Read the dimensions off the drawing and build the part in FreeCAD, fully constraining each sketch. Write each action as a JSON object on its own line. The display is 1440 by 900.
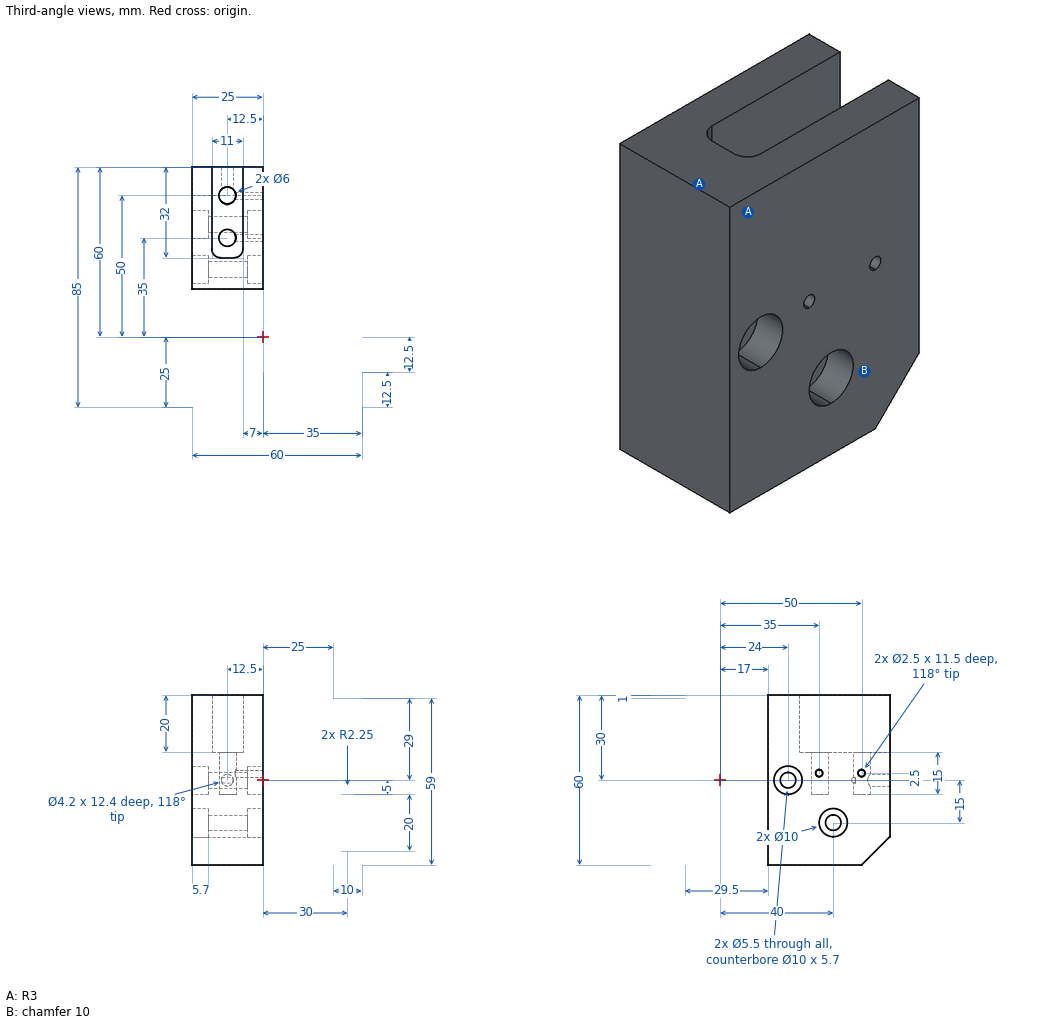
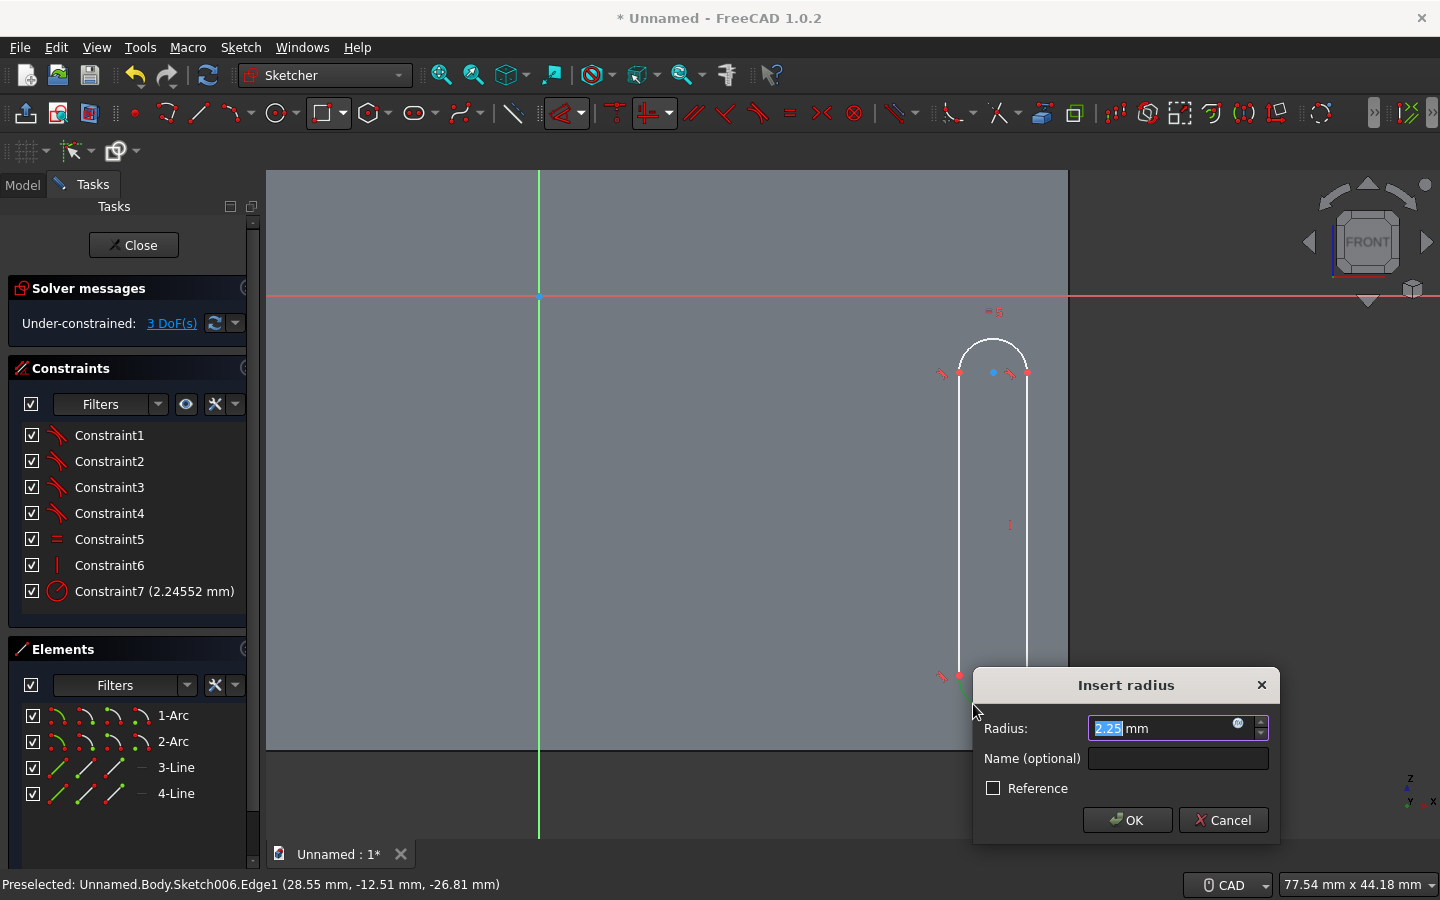
{"action": "type", "text": "2.25"}
{"action": "key", "text": "Return"}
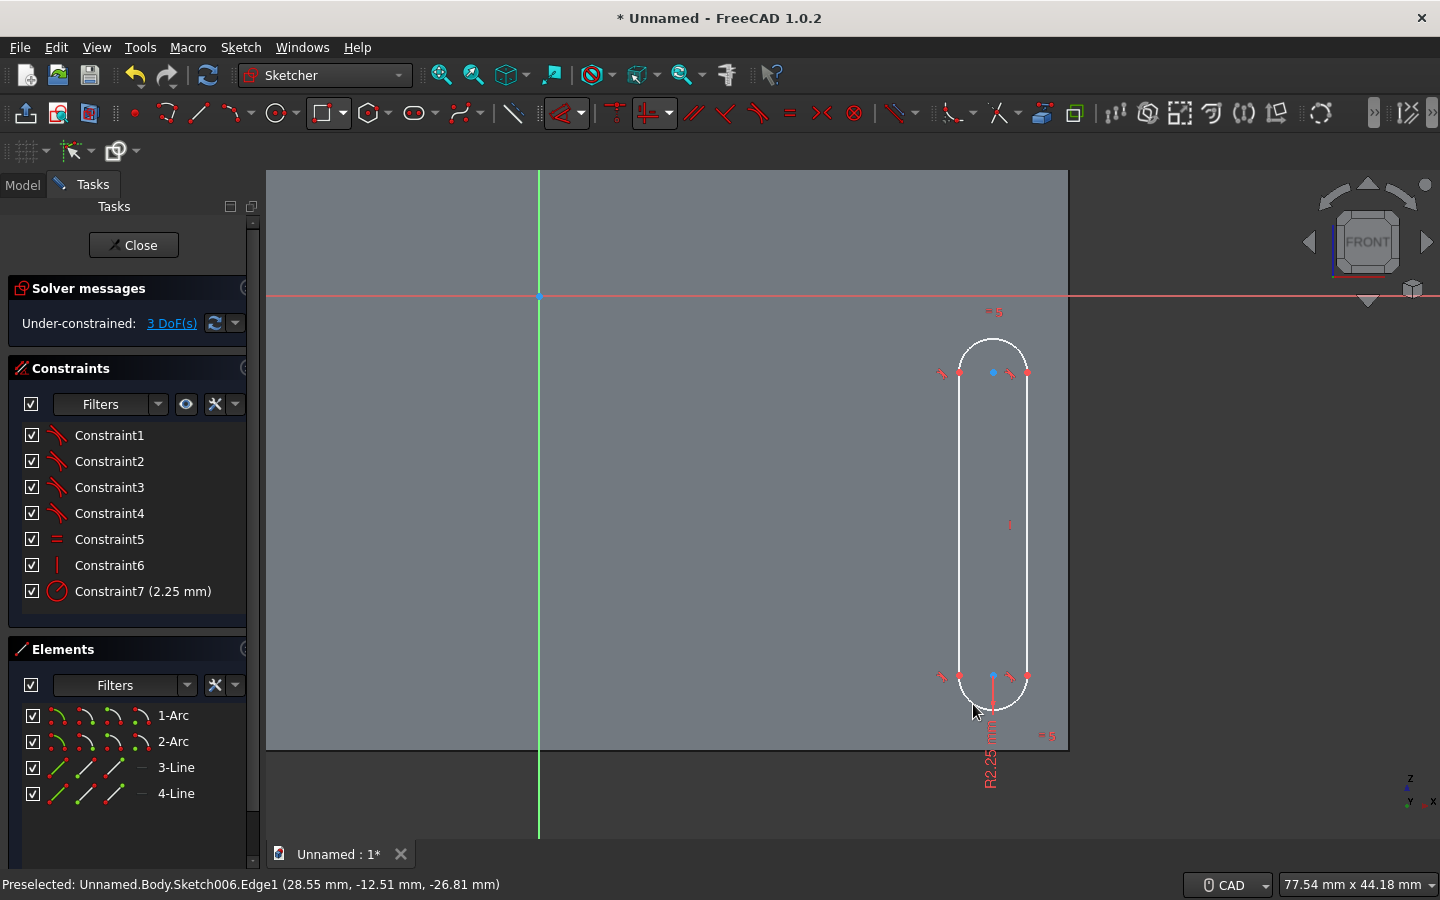
{"action": "left_click", "coordinate": [959, 585]}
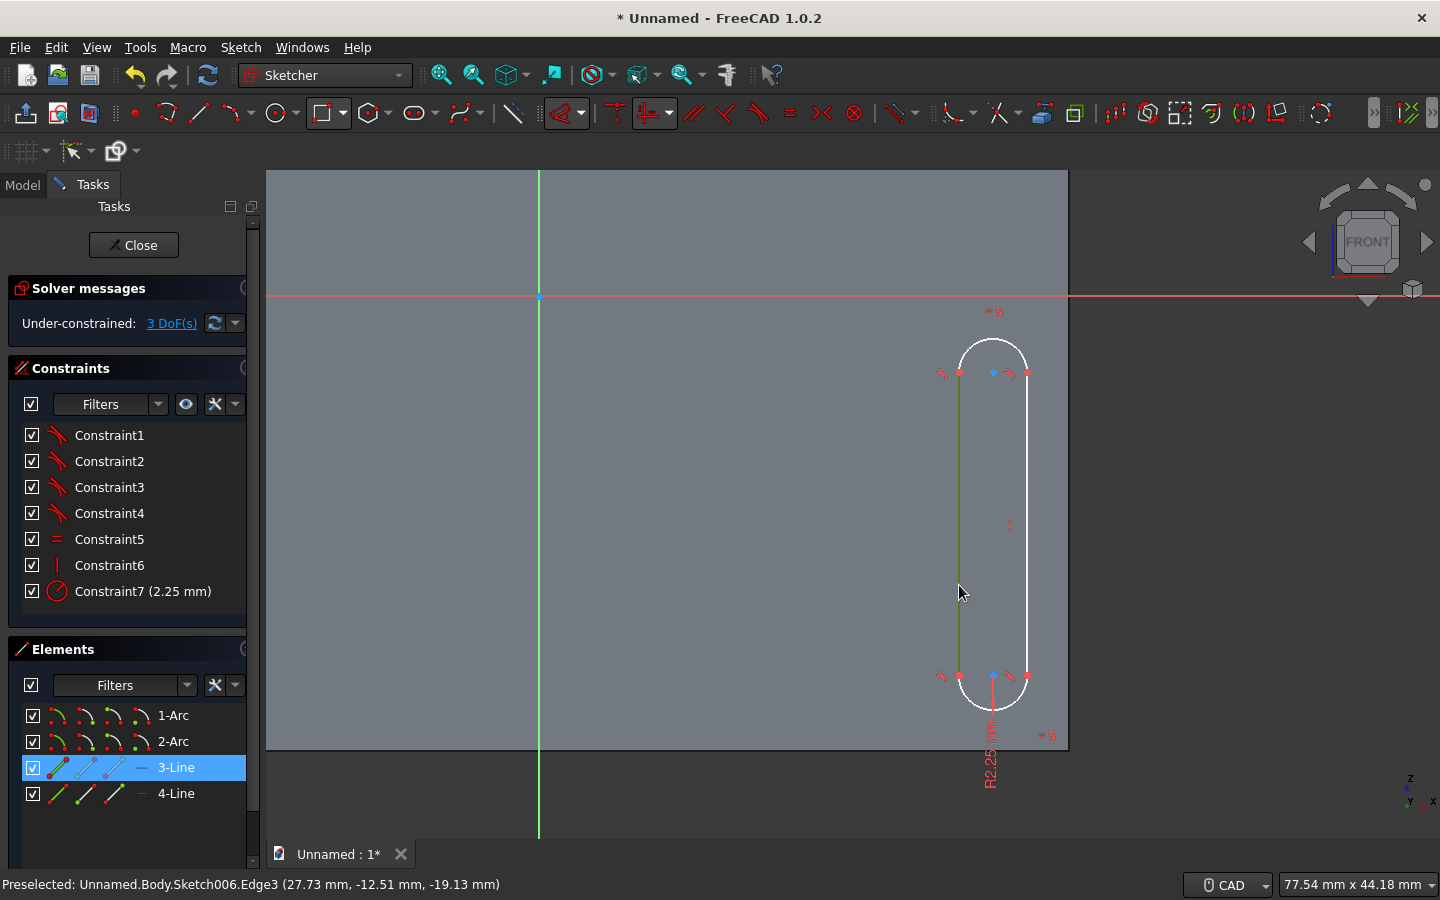
{"action": "key", "text": "i"}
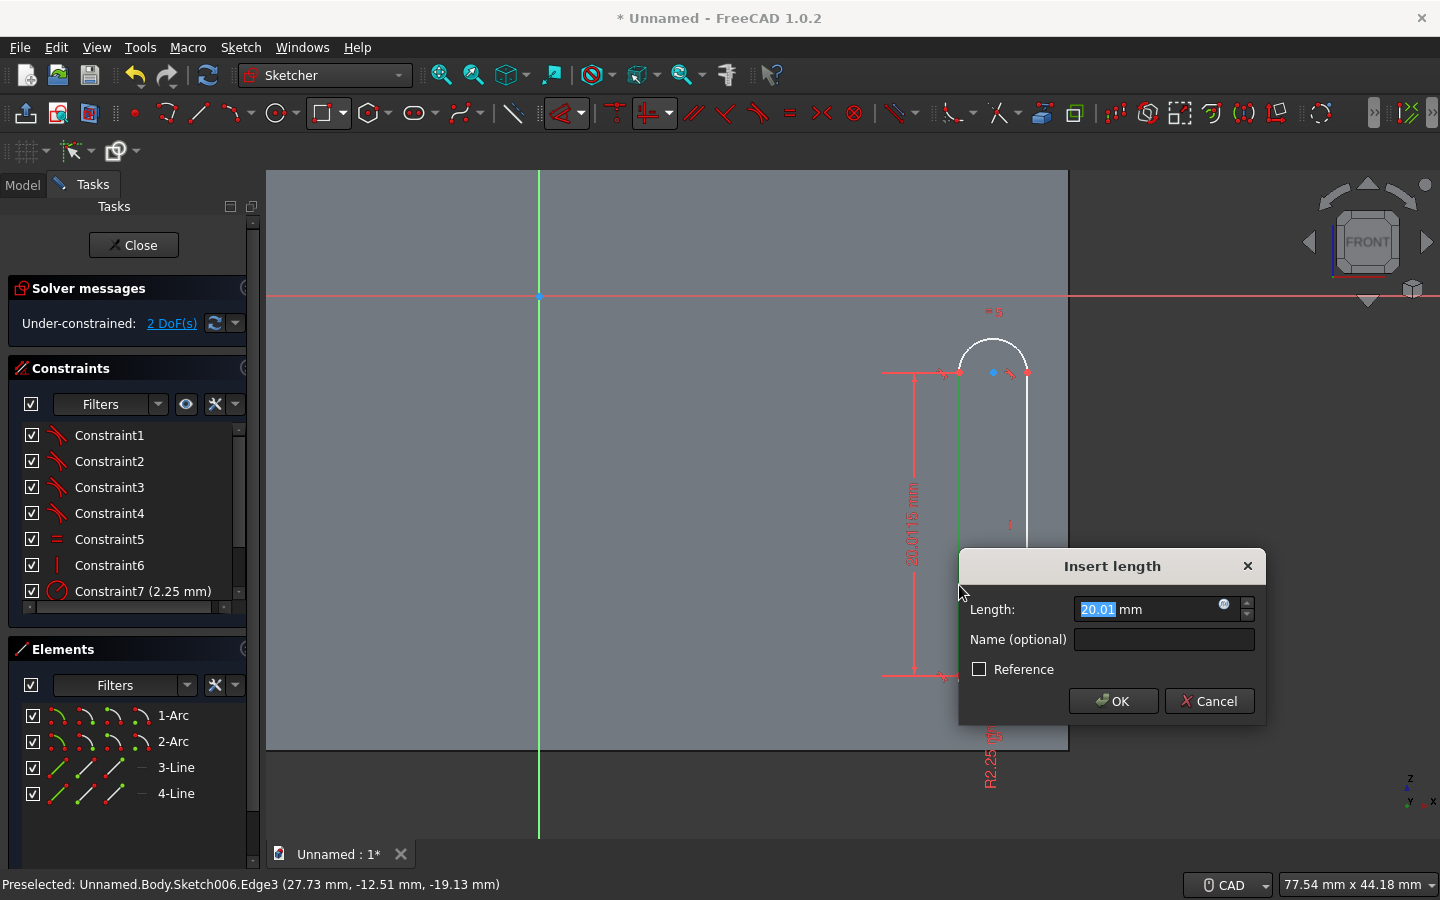
{"action": "type", "text": "20"}
{"action": "key", "text": "Return"}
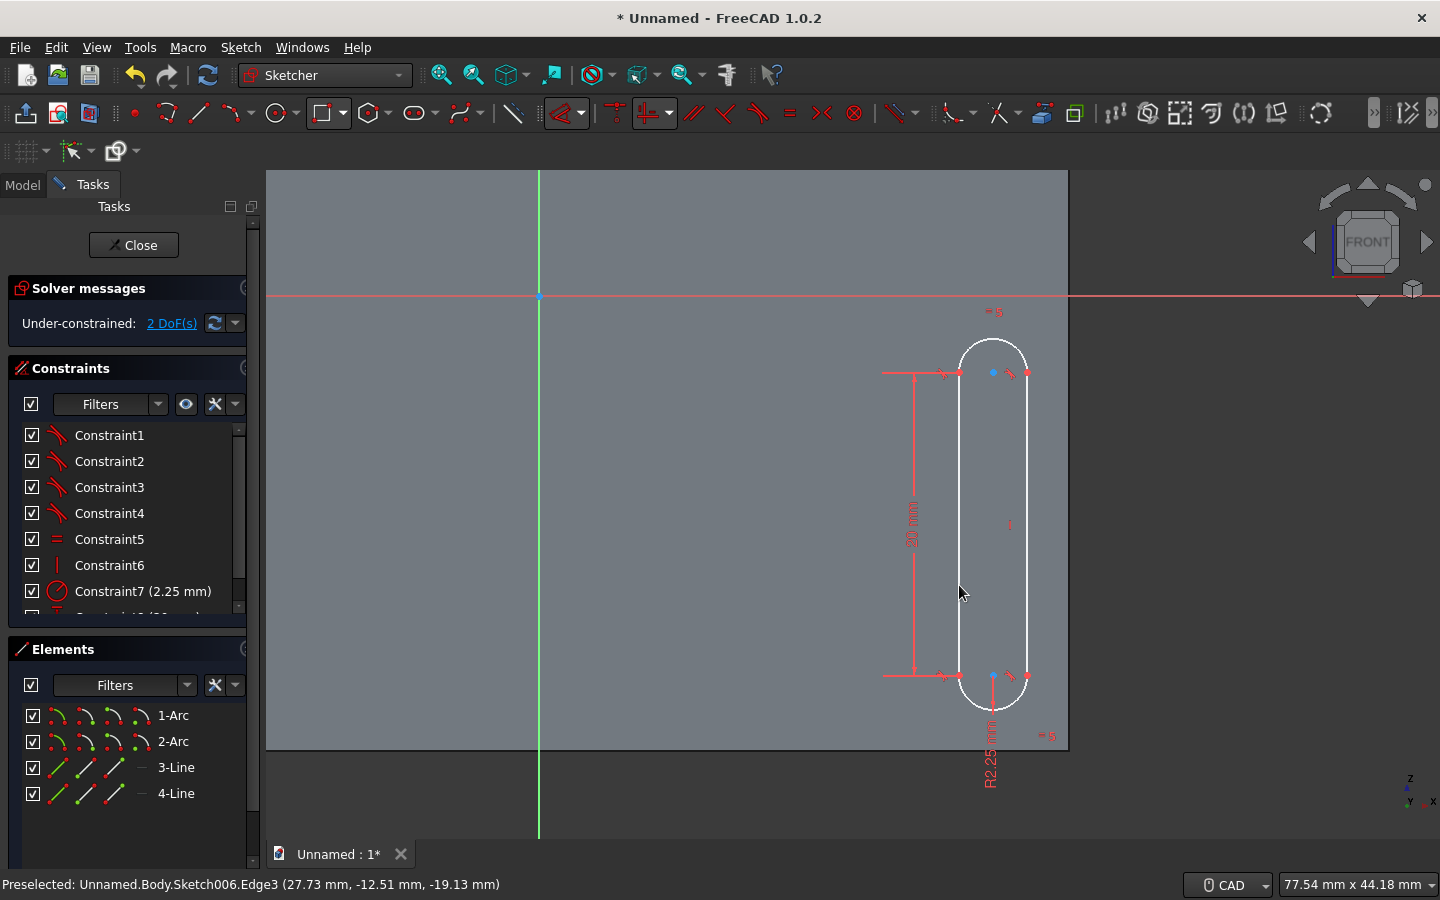
{"action": "left_click", "coordinate": [1027, 373]}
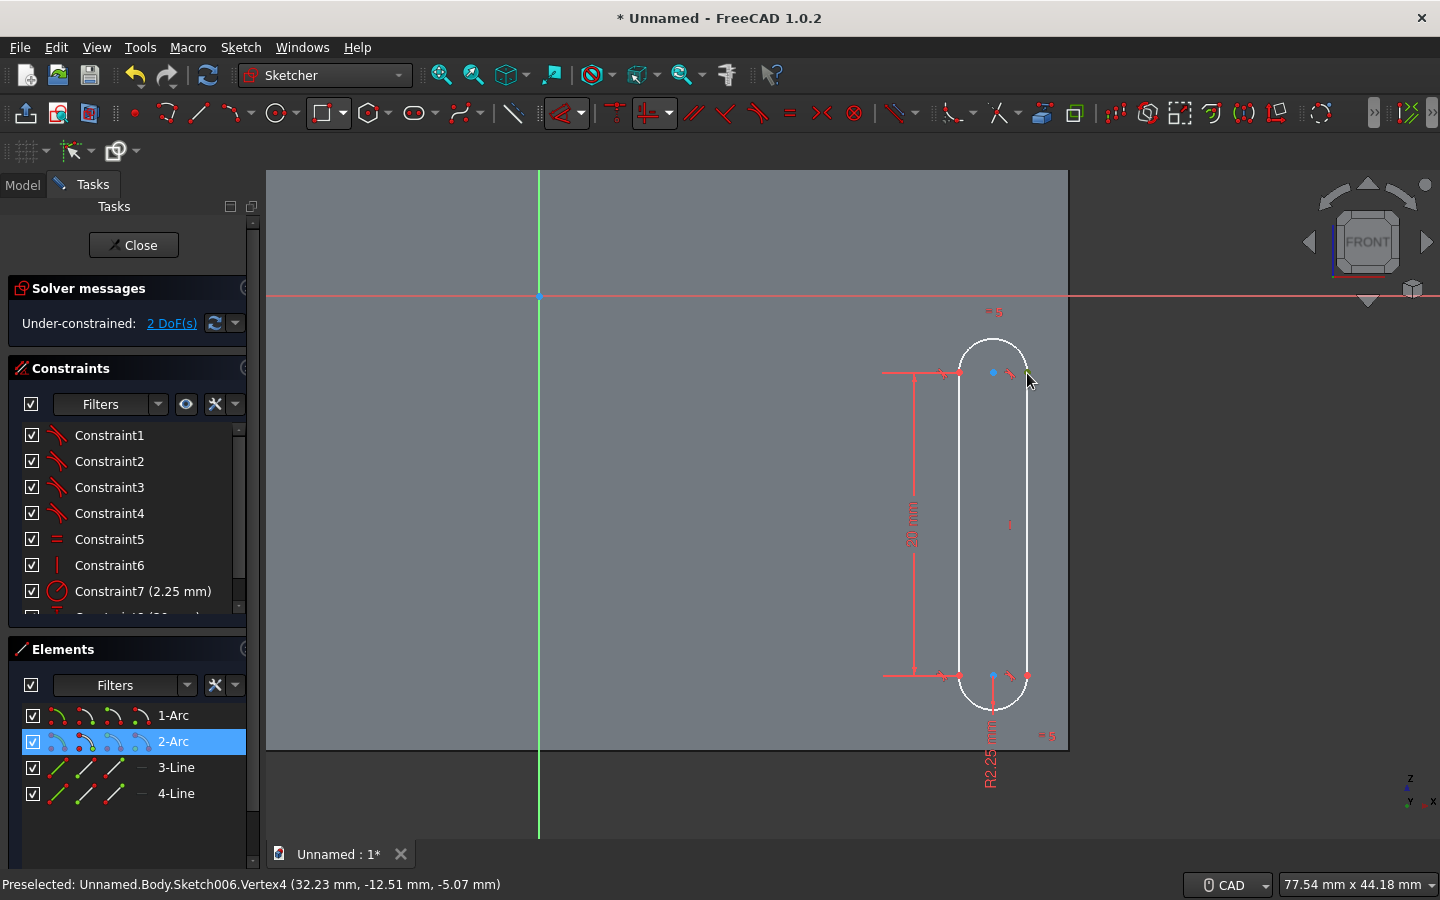
{"action": "left_click", "coordinate": [584, 114]}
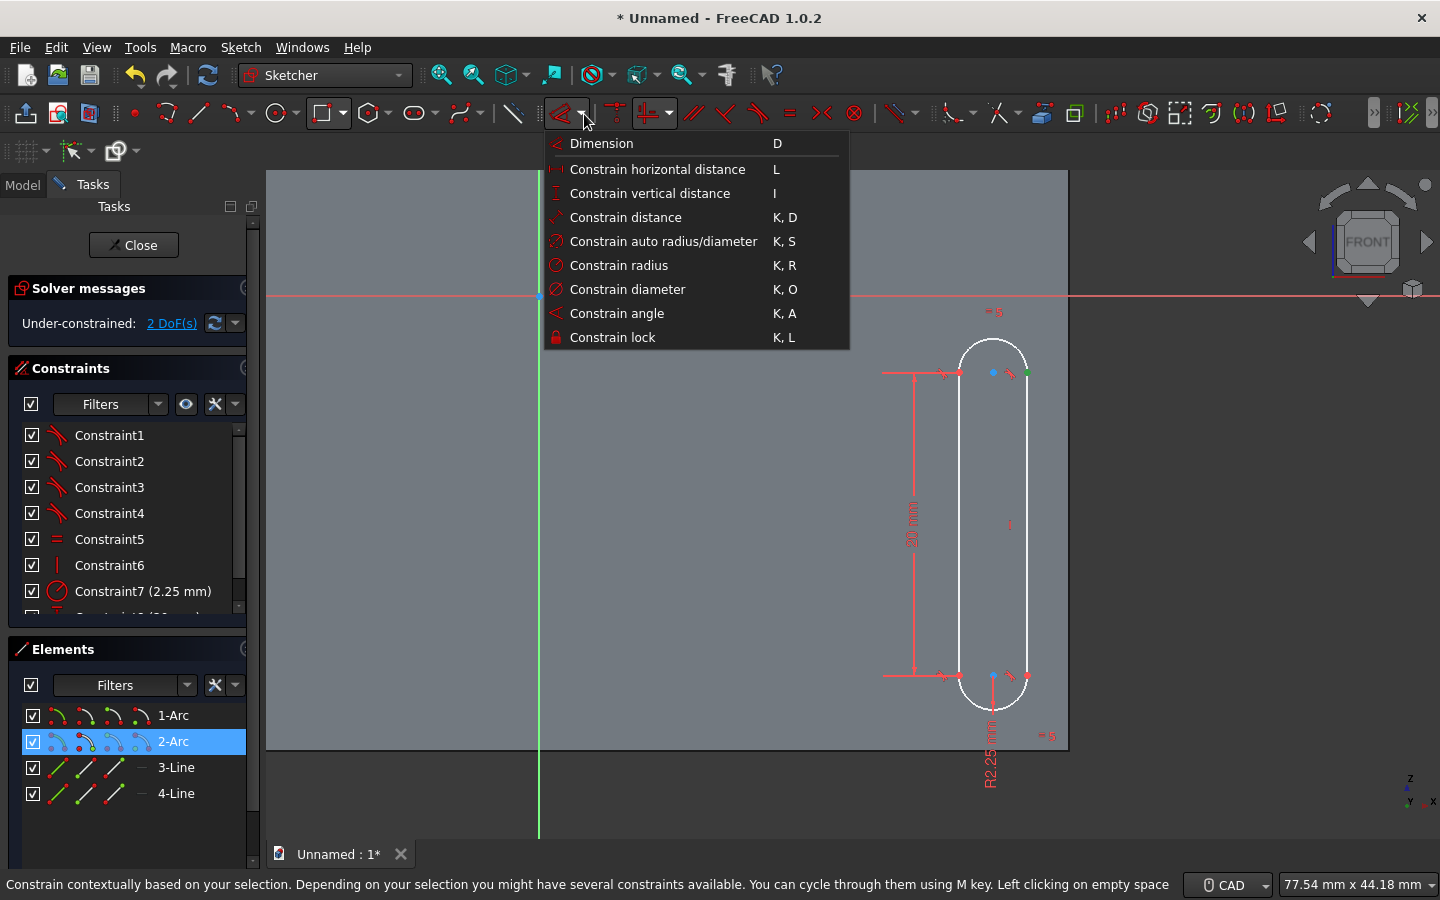
{"action": "left_click", "coordinate": [697, 193]}